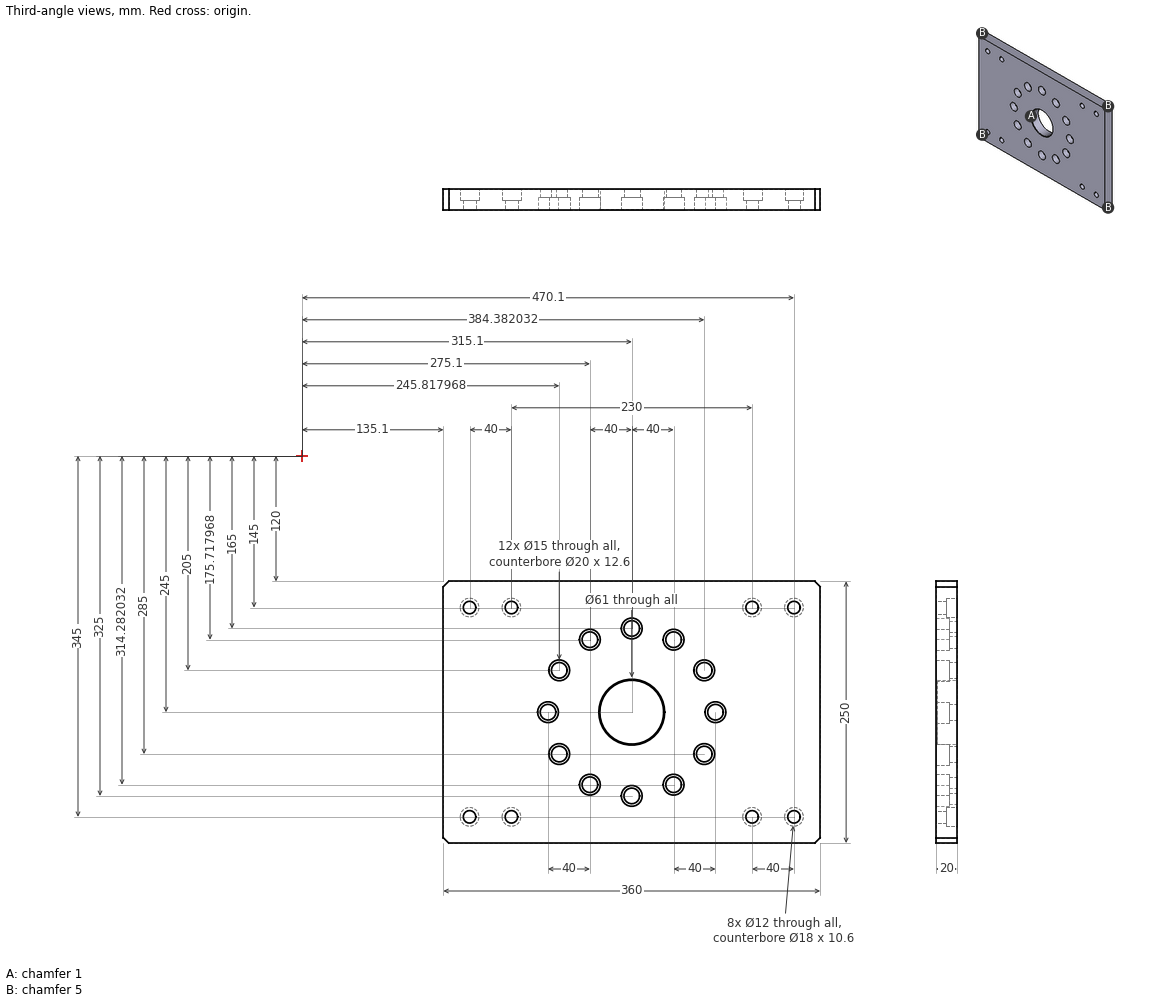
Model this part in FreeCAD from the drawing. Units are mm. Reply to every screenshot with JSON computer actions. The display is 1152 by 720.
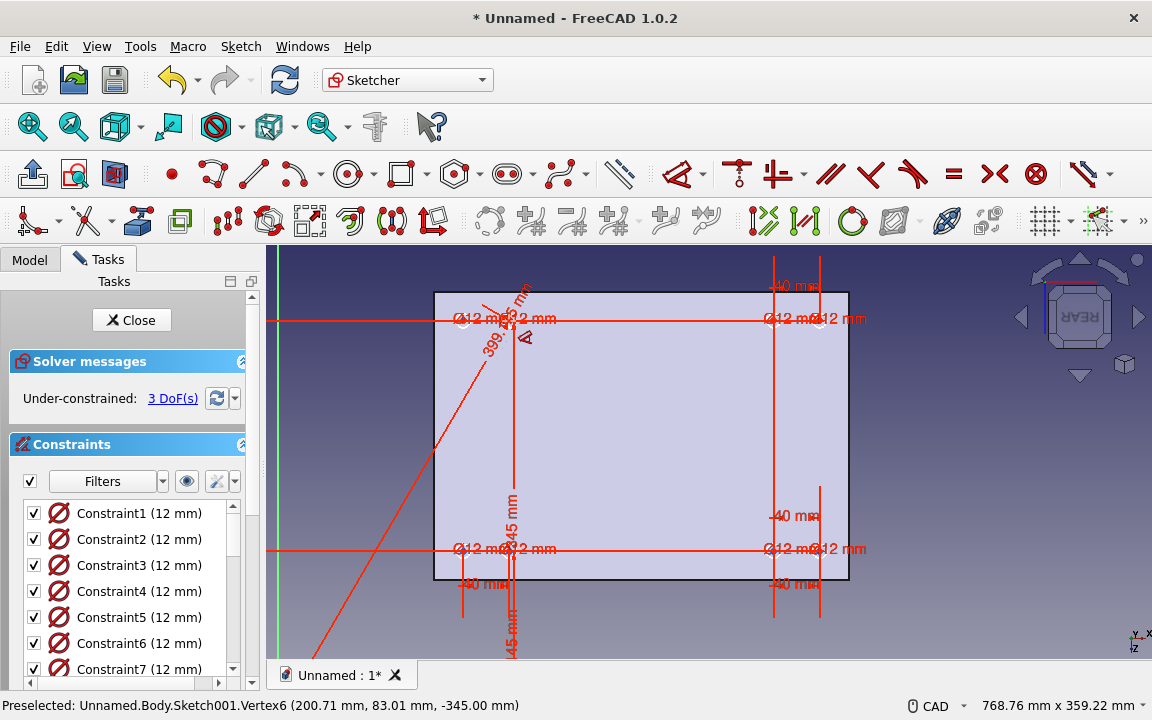
{"action": "left_click", "coordinate": [463, 551]}
{"action": "left_click", "coordinate": [486, 287]}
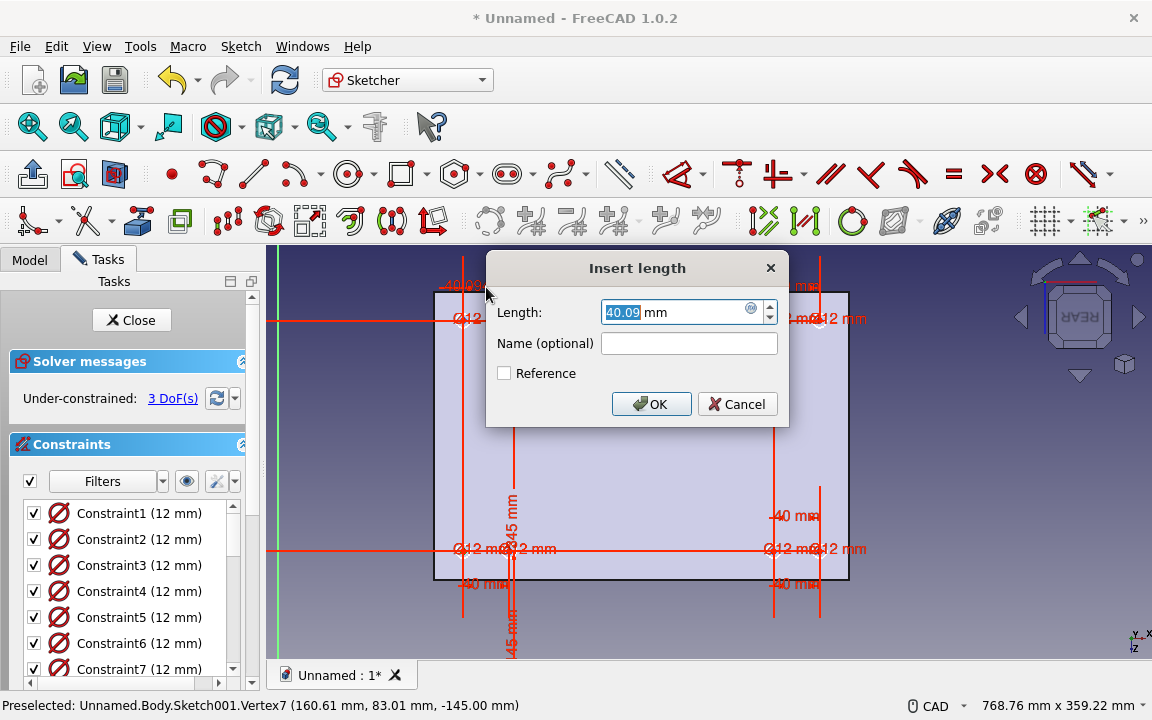
{"action": "type", "text": "40"}
{"action": "key", "text": "Return"}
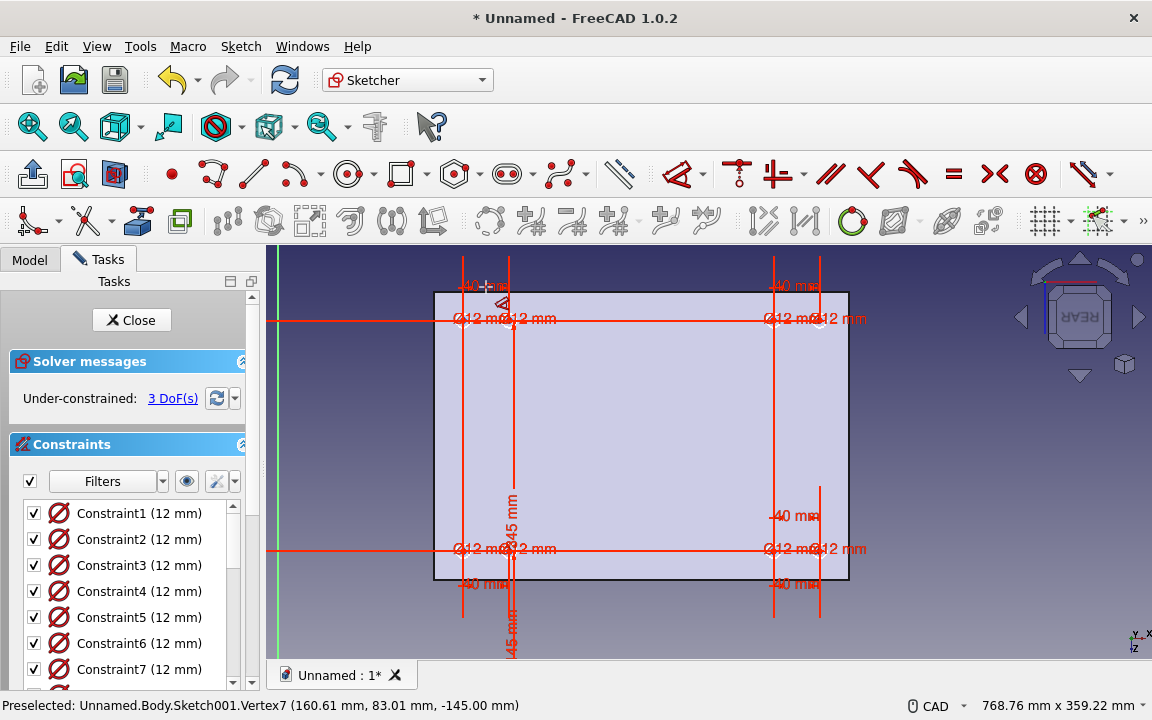
{"action": "left_click", "coordinate": [509, 321]}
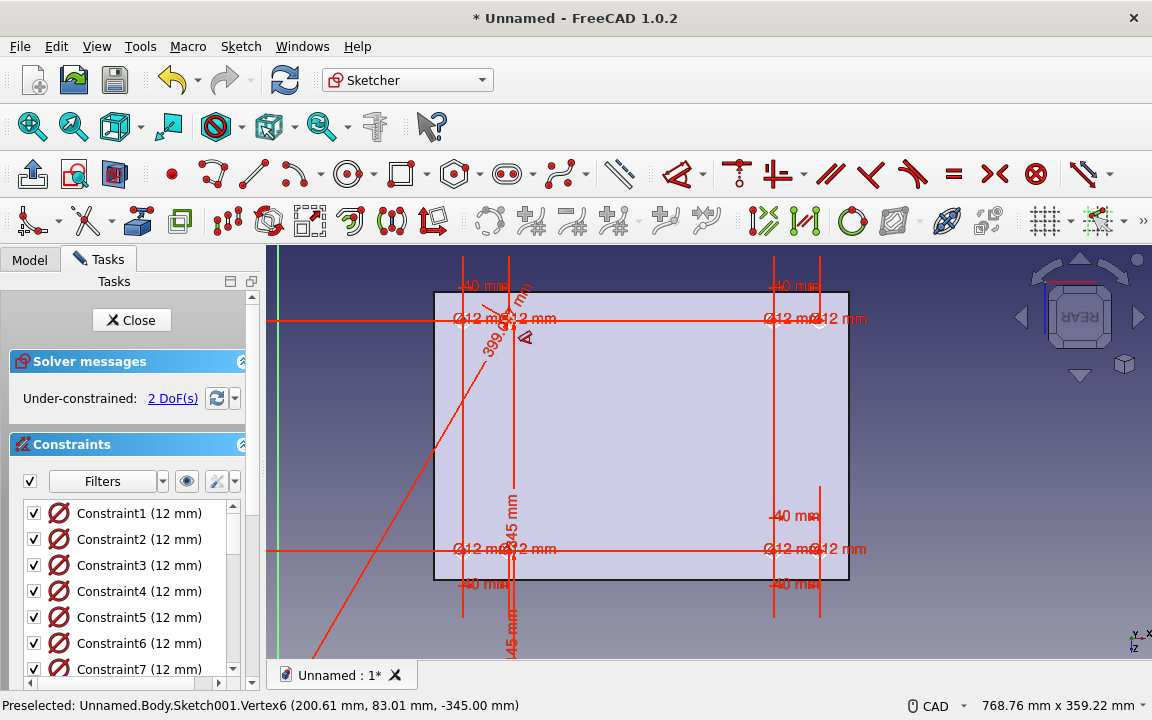
{"action": "left_click", "coordinate": [463, 321]}
{"action": "left_click", "coordinate": [486, 355]}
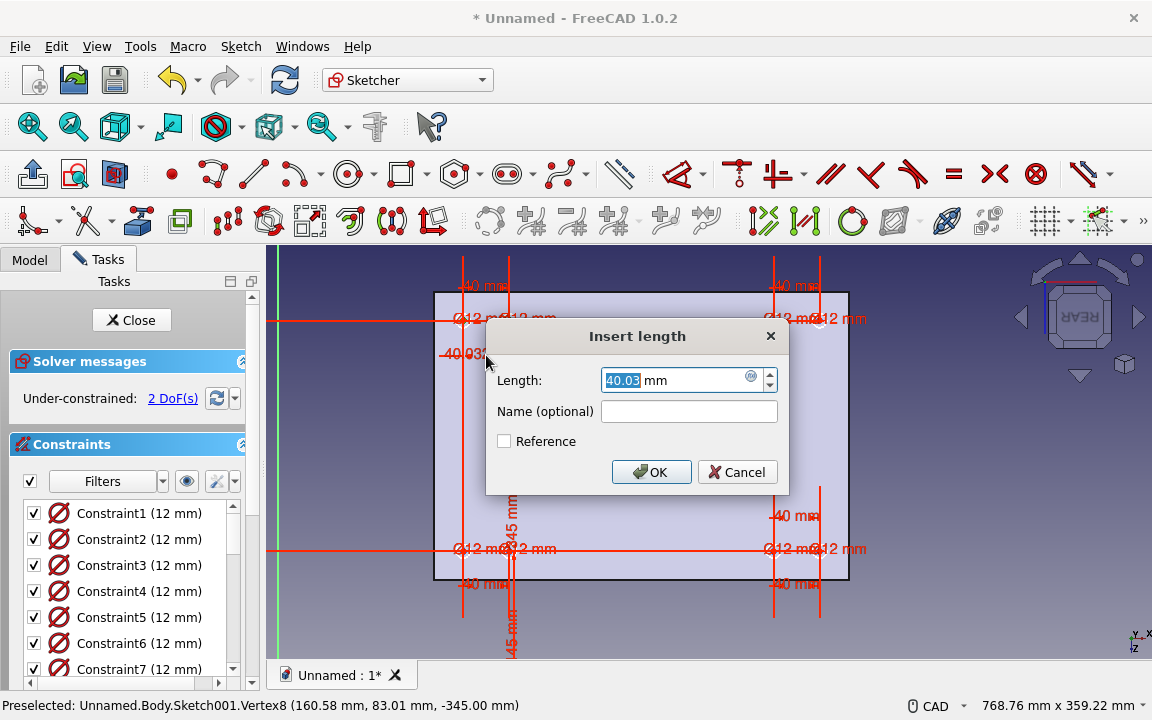
{"action": "type", "text": "40"}
{"action": "key", "text": "Return"}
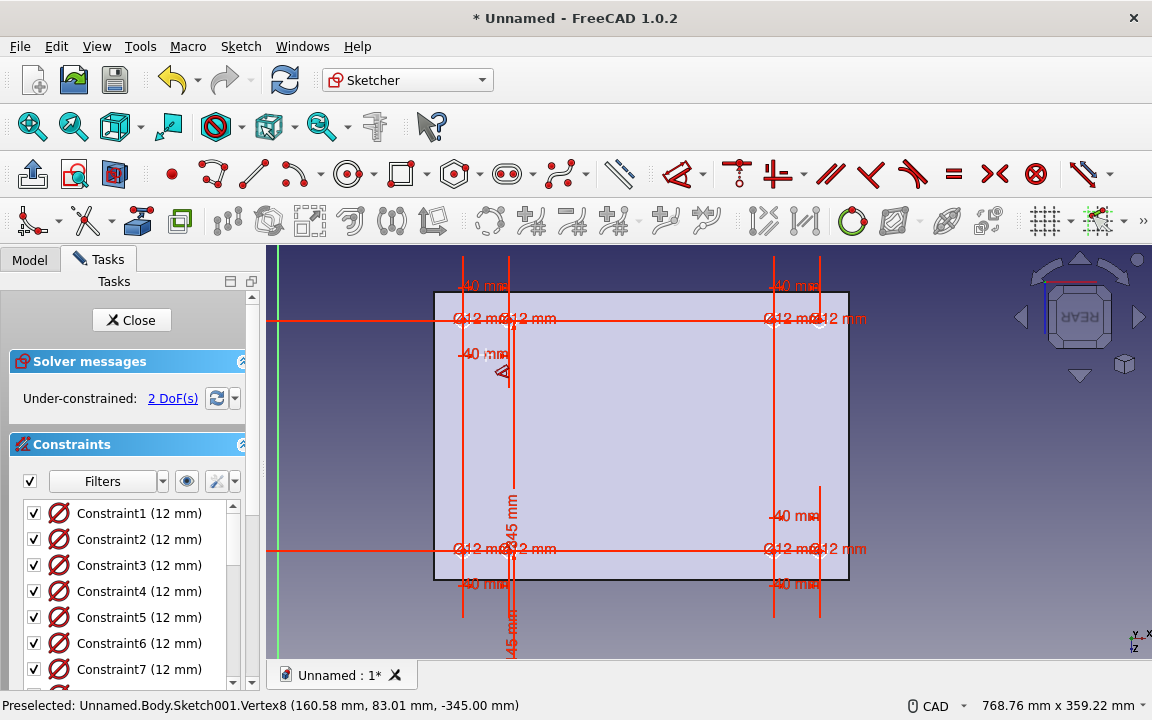
{"action": "left_click", "coordinate": [774, 551]}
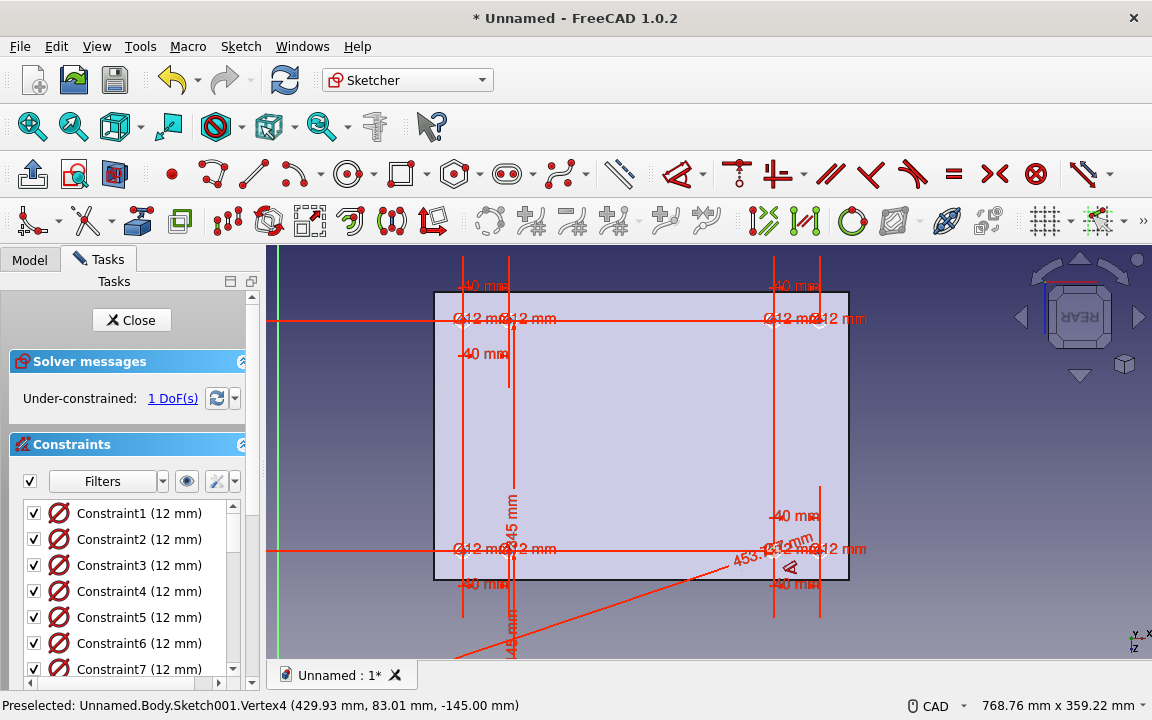
{"action": "left_click", "coordinate": [509, 551]}
{"action": "left_click", "coordinate": [641, 585]}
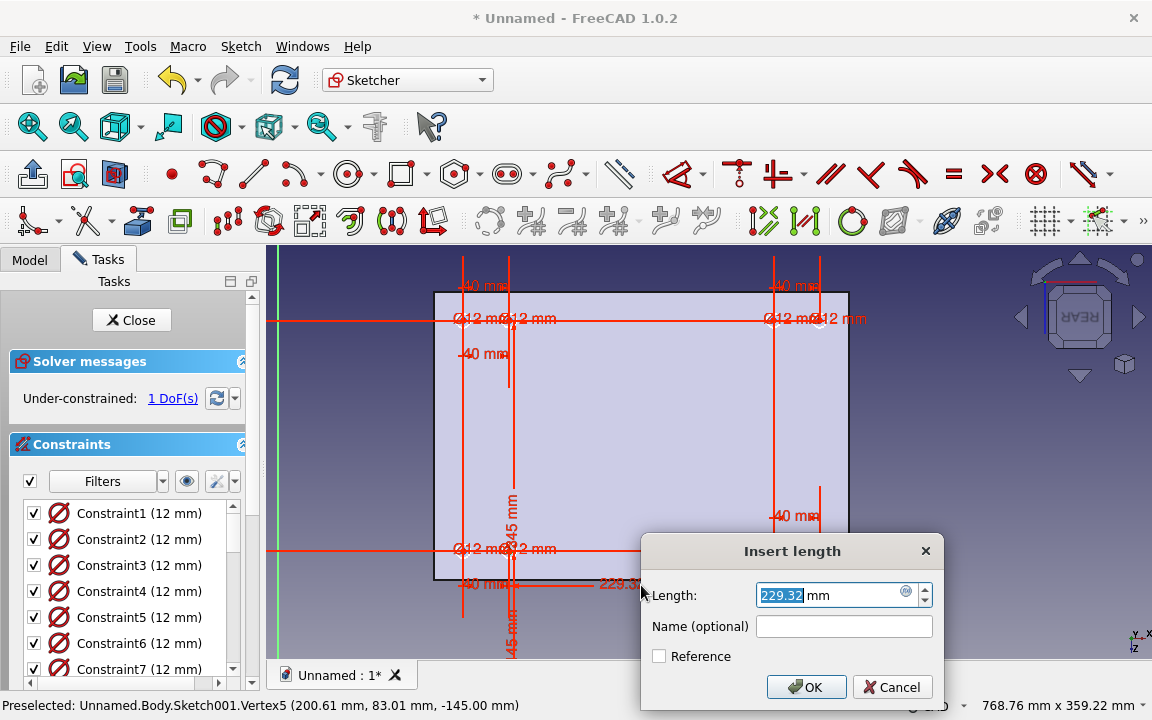
{"action": "type", "text": "230"}
{"action": "key", "text": "Return"}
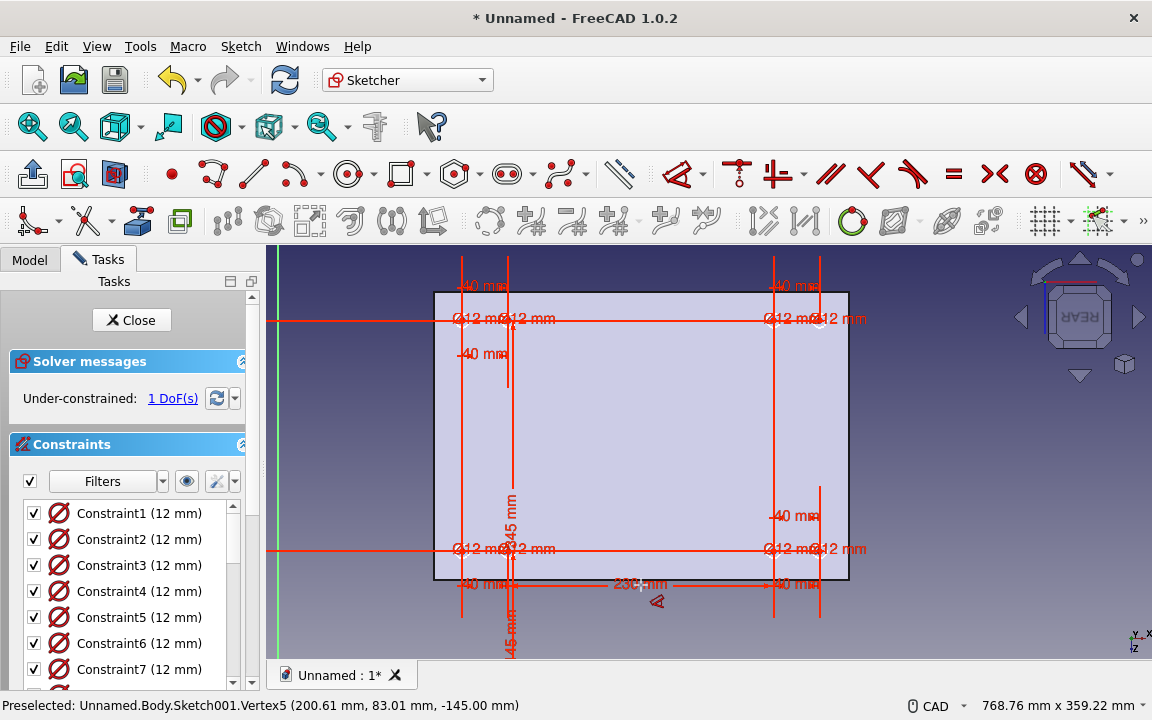
{"action": "left_click", "coordinate": [820, 321]}
{"action": "left_click", "coordinate": [557, 287]}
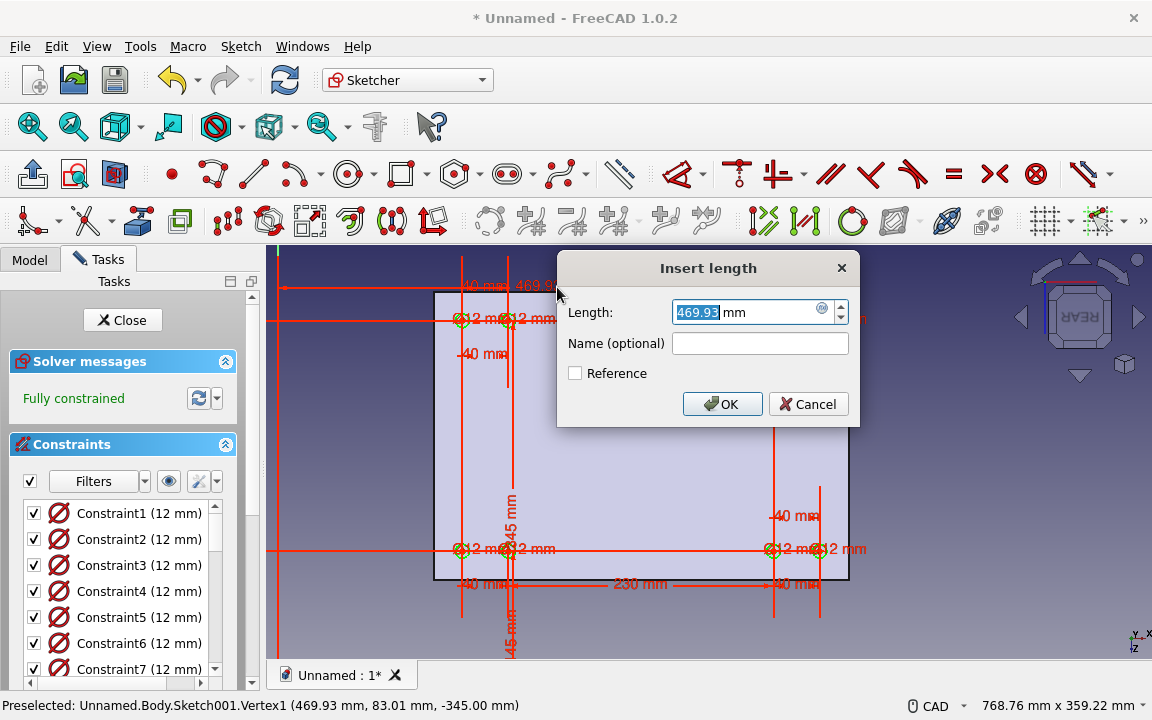
{"action": "type", "text": "470.1"}
{"action": "key", "text": "Return"}
{"action": "key", "text": "Escape"}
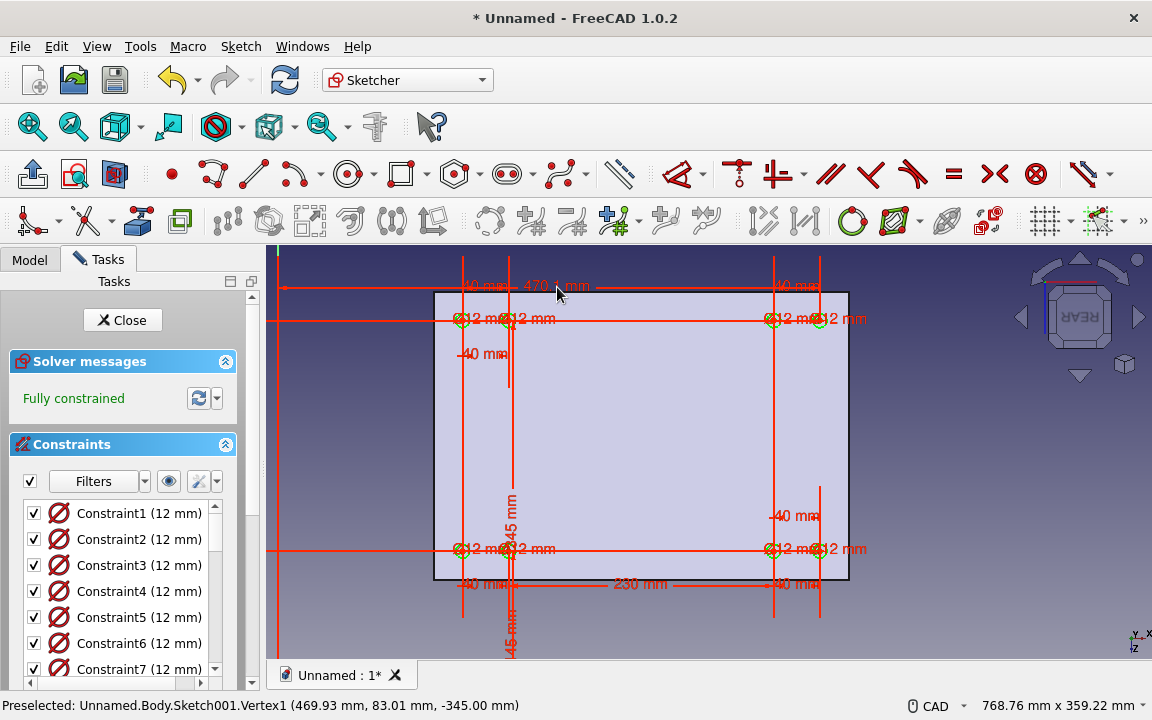
{"action": "left_click", "coordinate": [123, 320]}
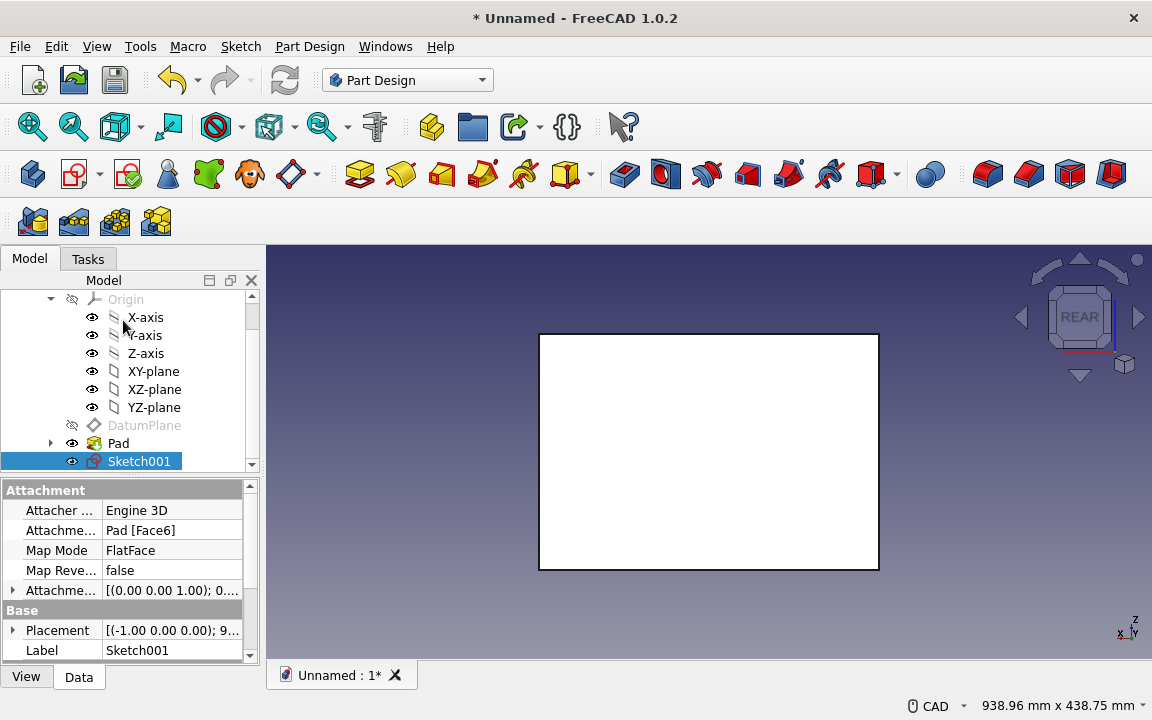
{"action": "left_click", "coordinate": [666, 174]}